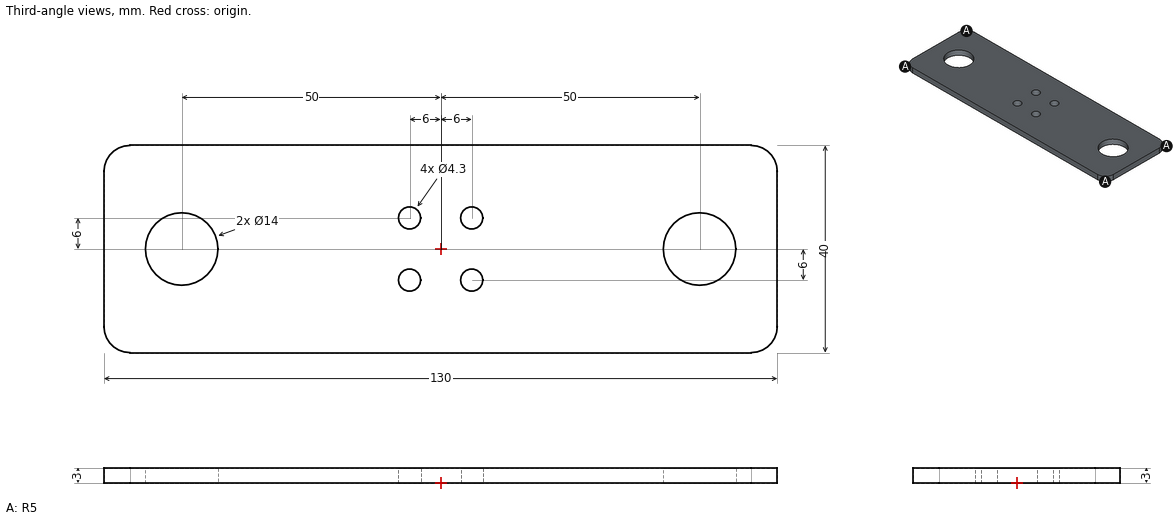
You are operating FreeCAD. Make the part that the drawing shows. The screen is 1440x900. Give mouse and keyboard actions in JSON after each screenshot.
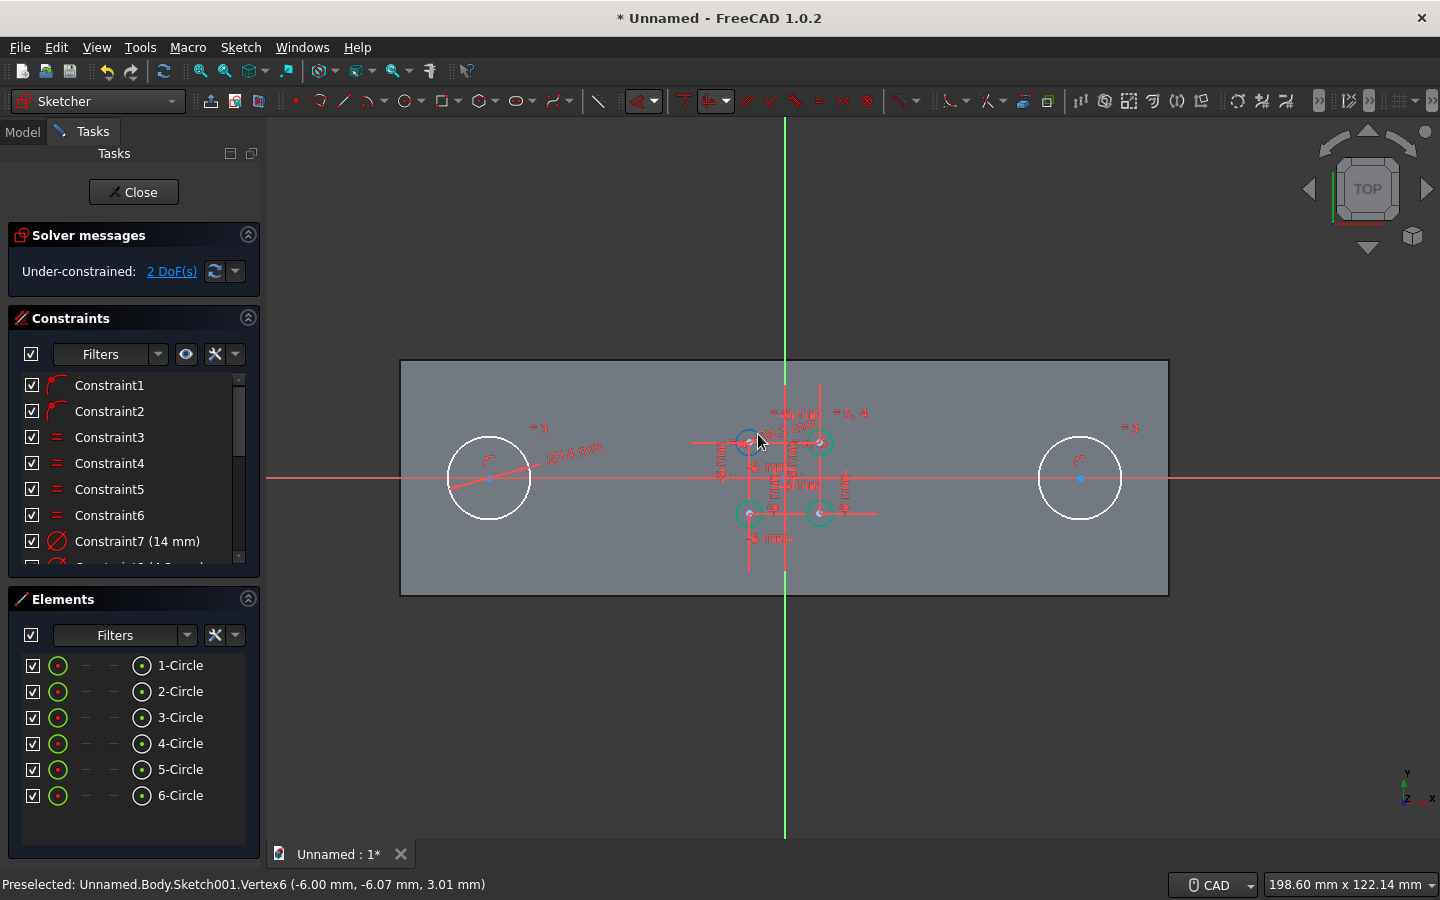
{"action": "left_click", "coordinate": [489, 478]}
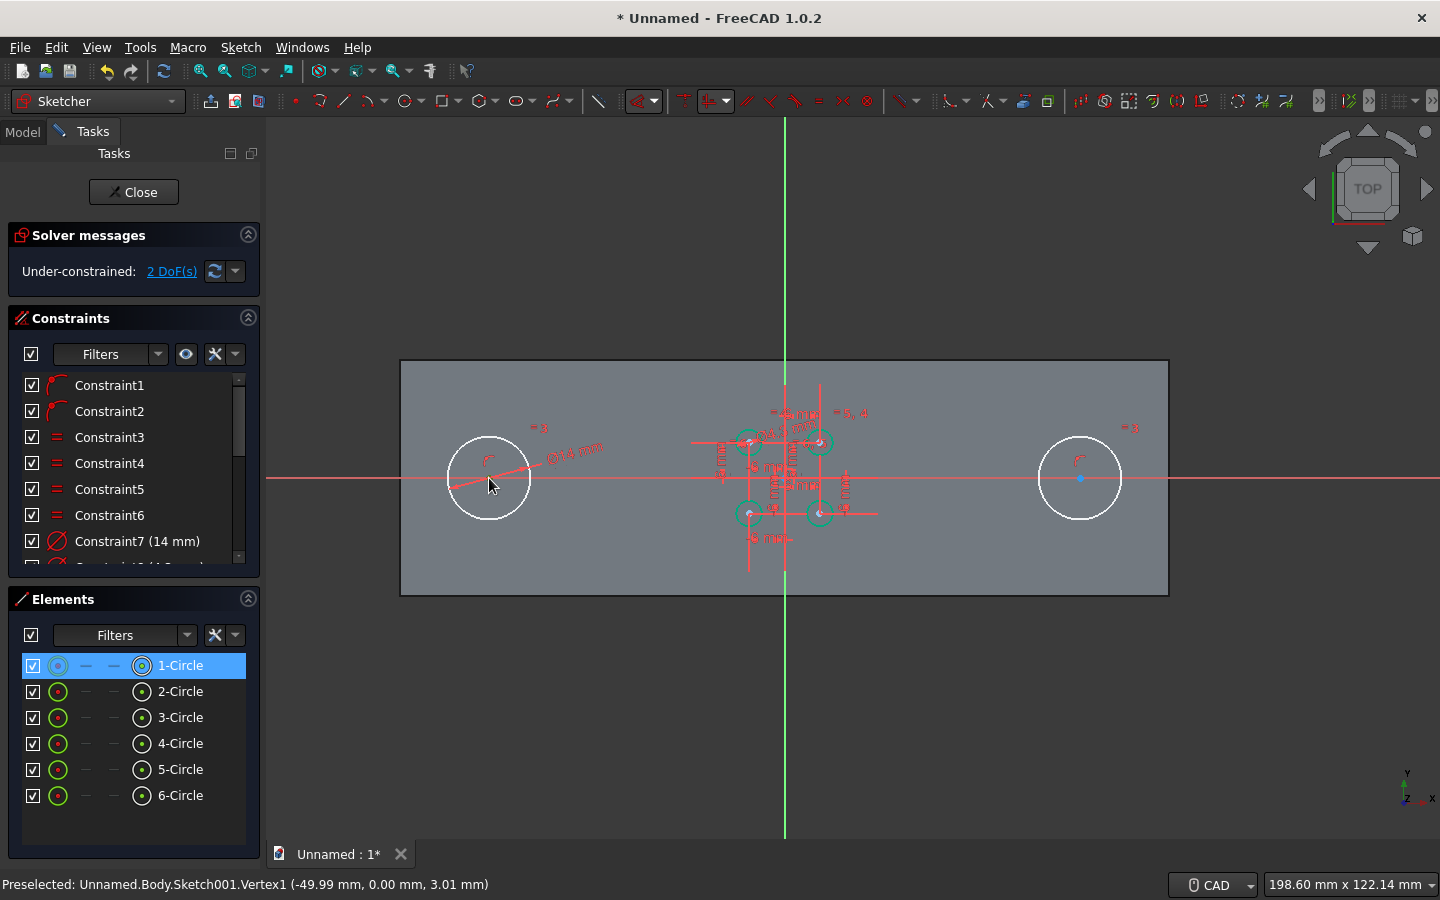
{"action": "key", "text": "l"}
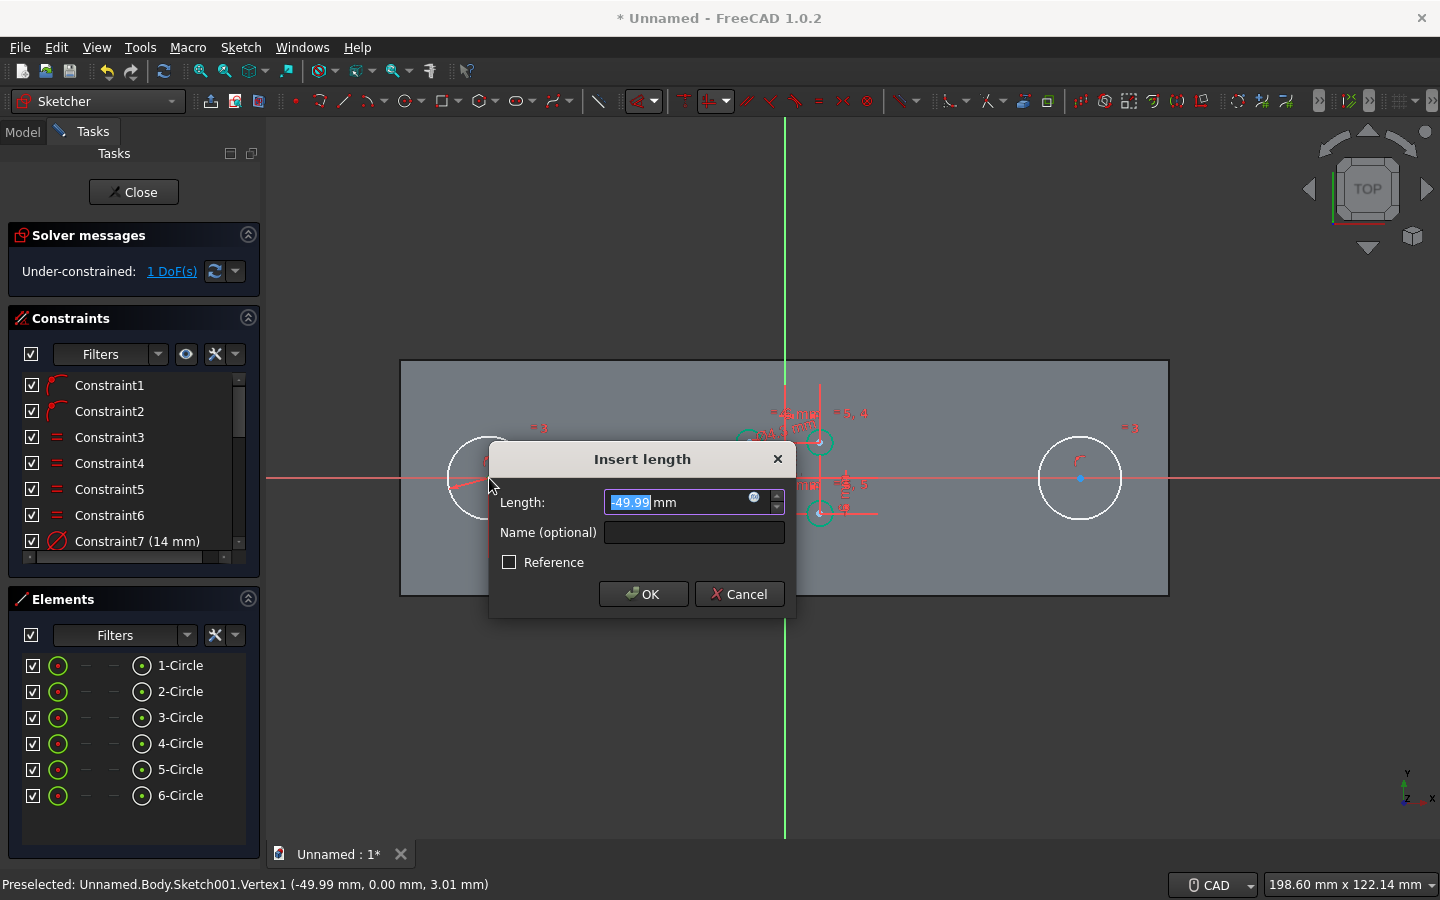
{"action": "type", "text": "-50"}
{"action": "key", "text": "Return"}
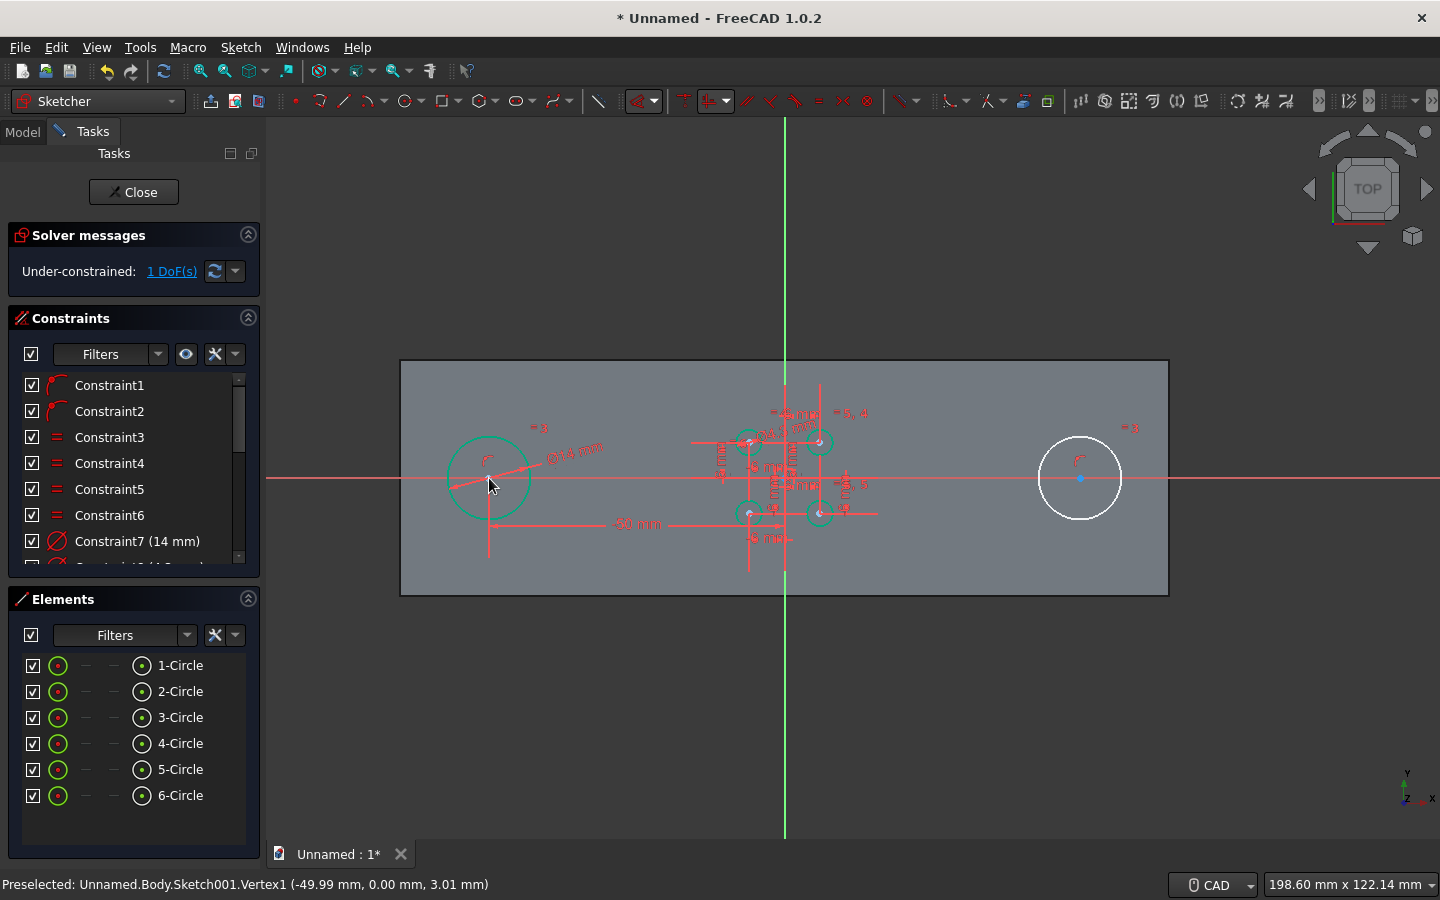
{"action": "left_click", "coordinate": [1080, 478]}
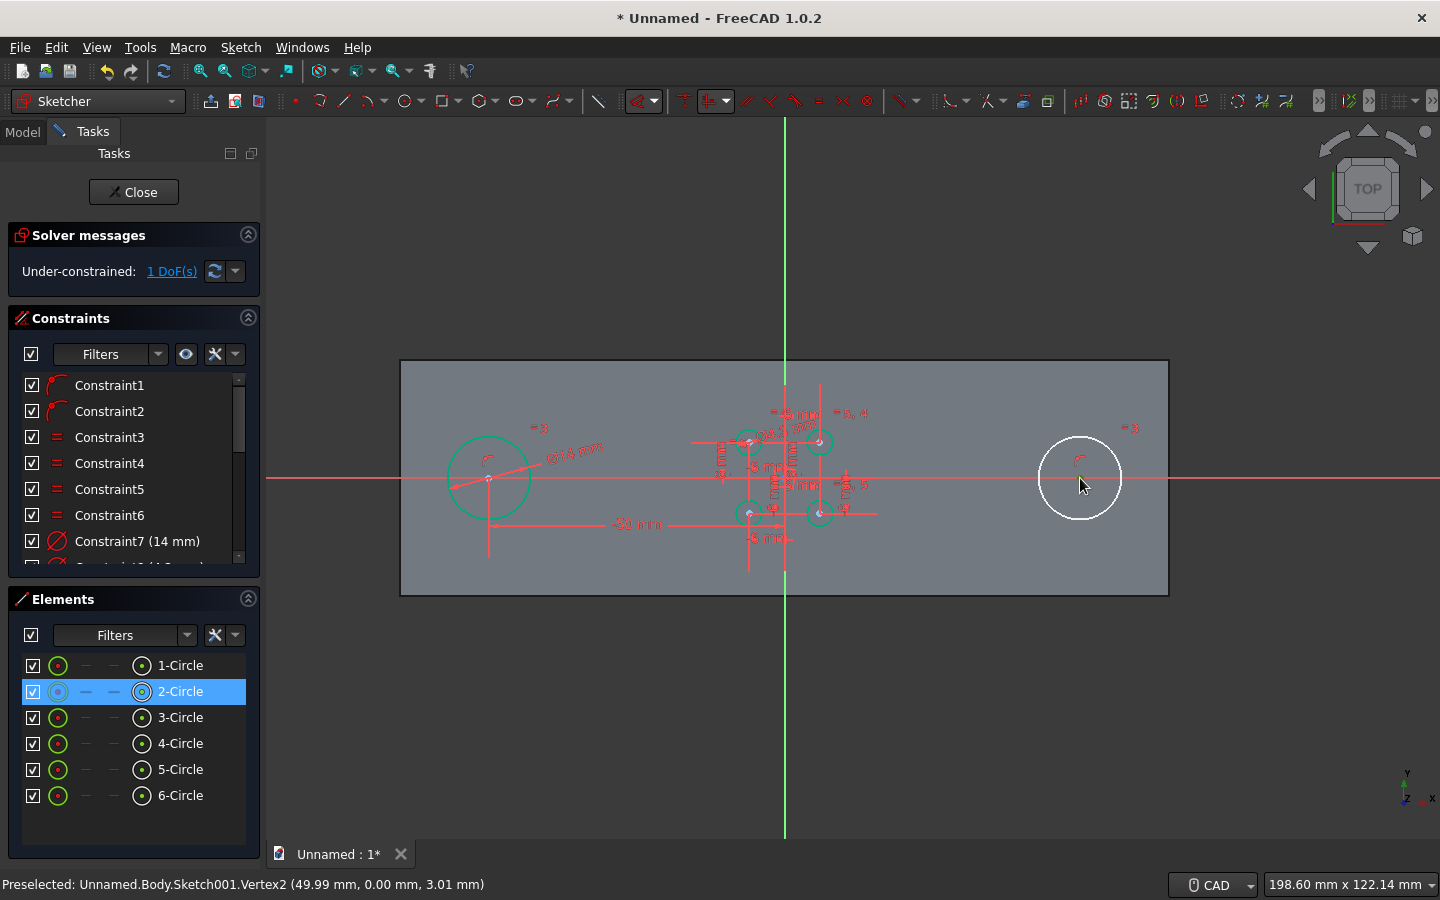
{"action": "key", "text": "l"}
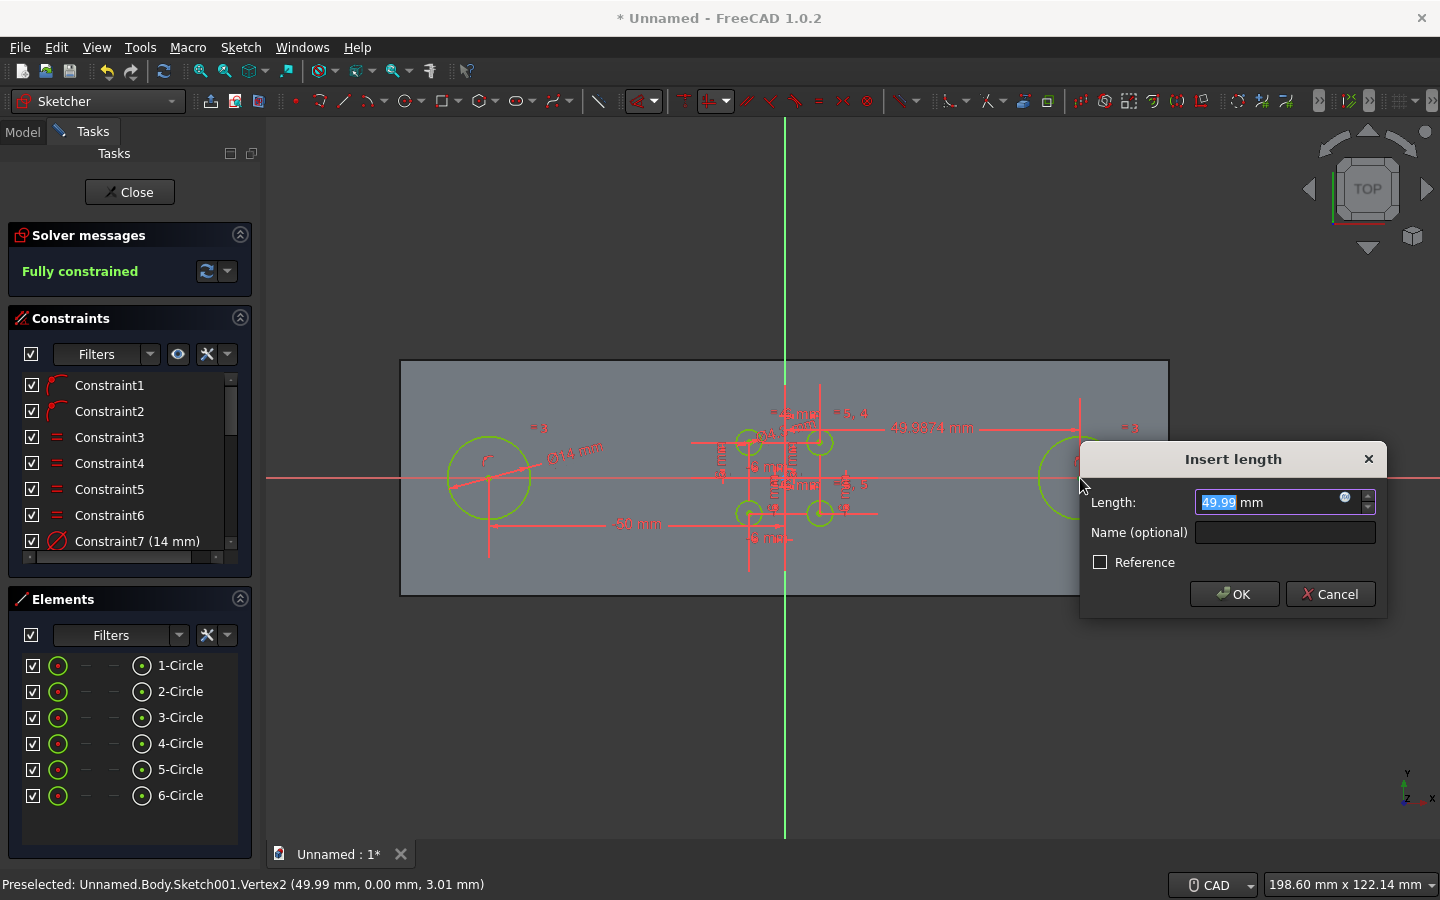
{"action": "type", "text": "50"}
{"action": "key", "text": "Return"}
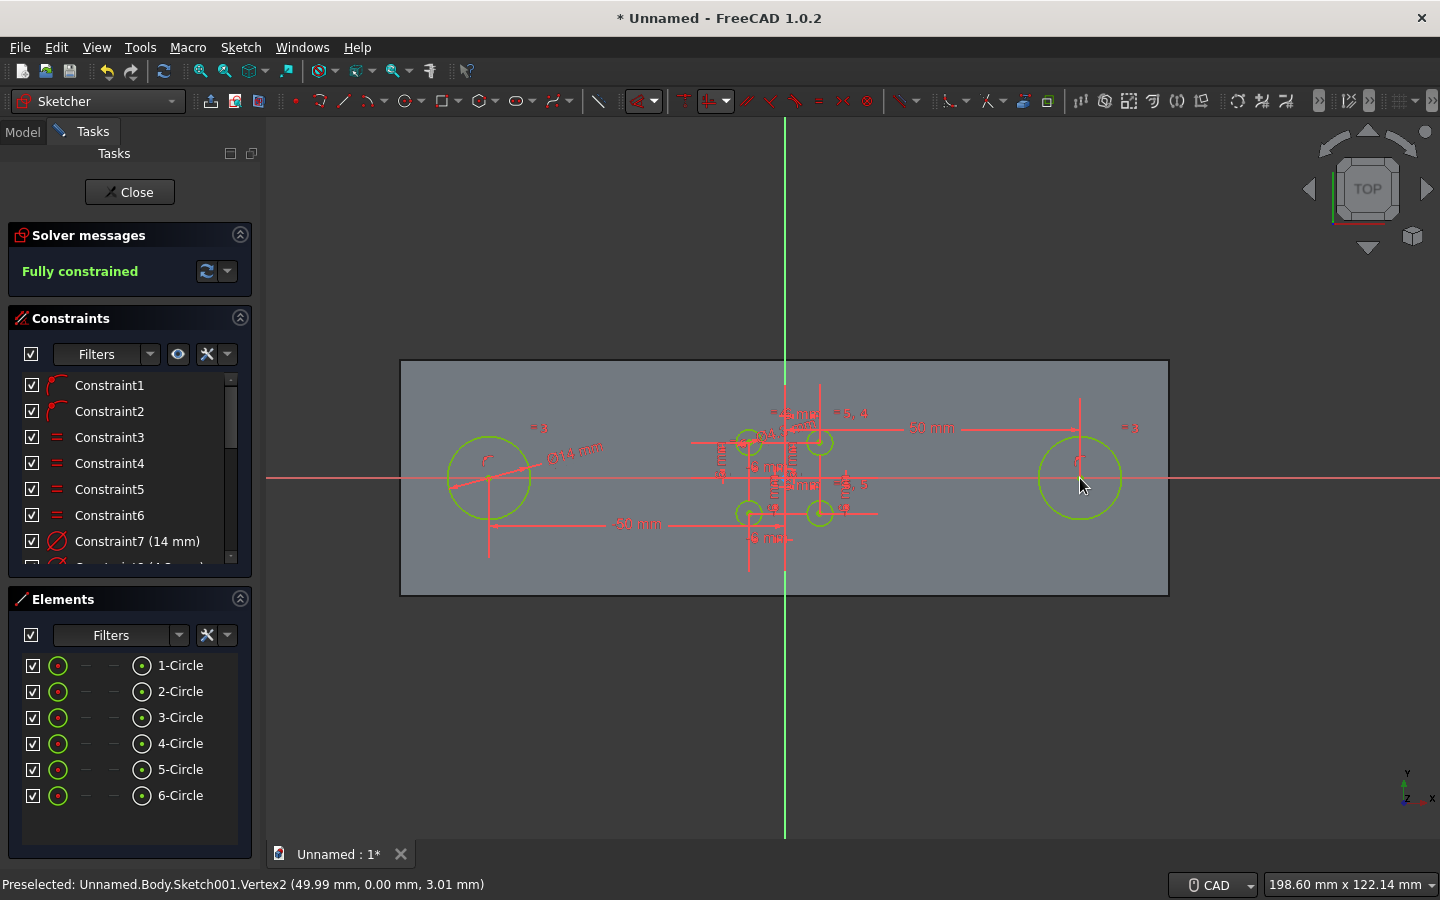
{"action": "left_click", "coordinate": [130, 192]}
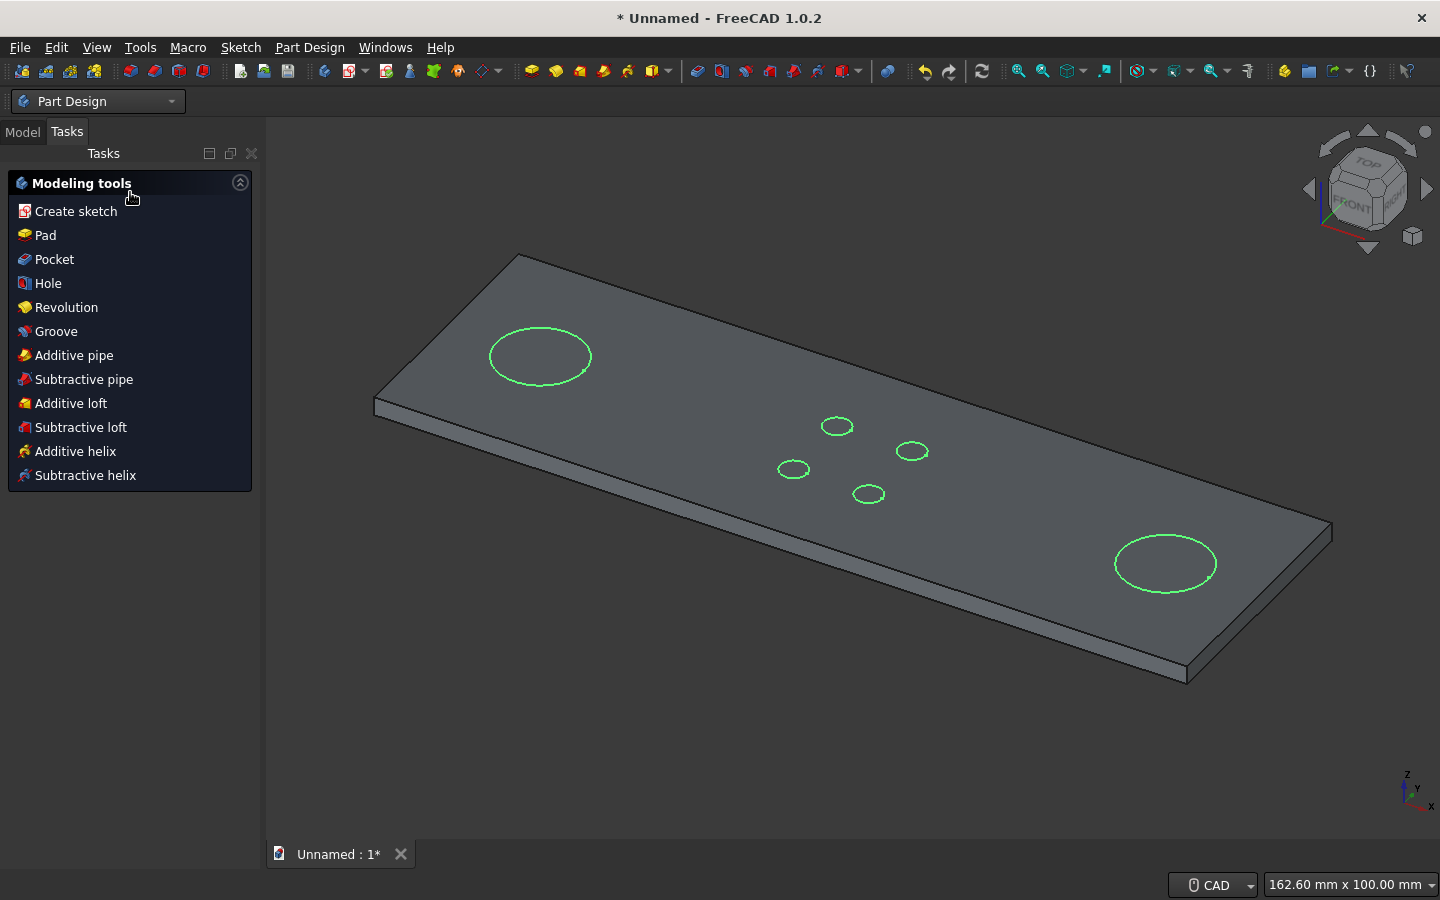
{"action": "left_click", "coordinate": [698, 72]}